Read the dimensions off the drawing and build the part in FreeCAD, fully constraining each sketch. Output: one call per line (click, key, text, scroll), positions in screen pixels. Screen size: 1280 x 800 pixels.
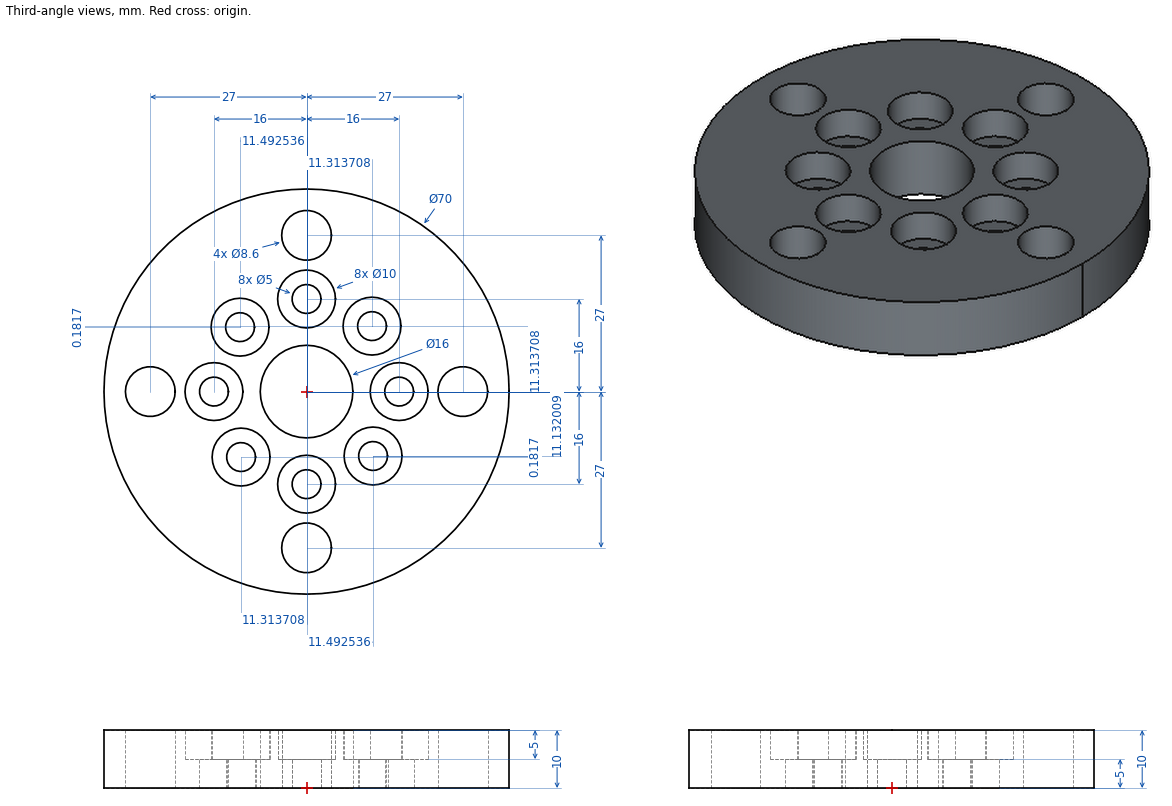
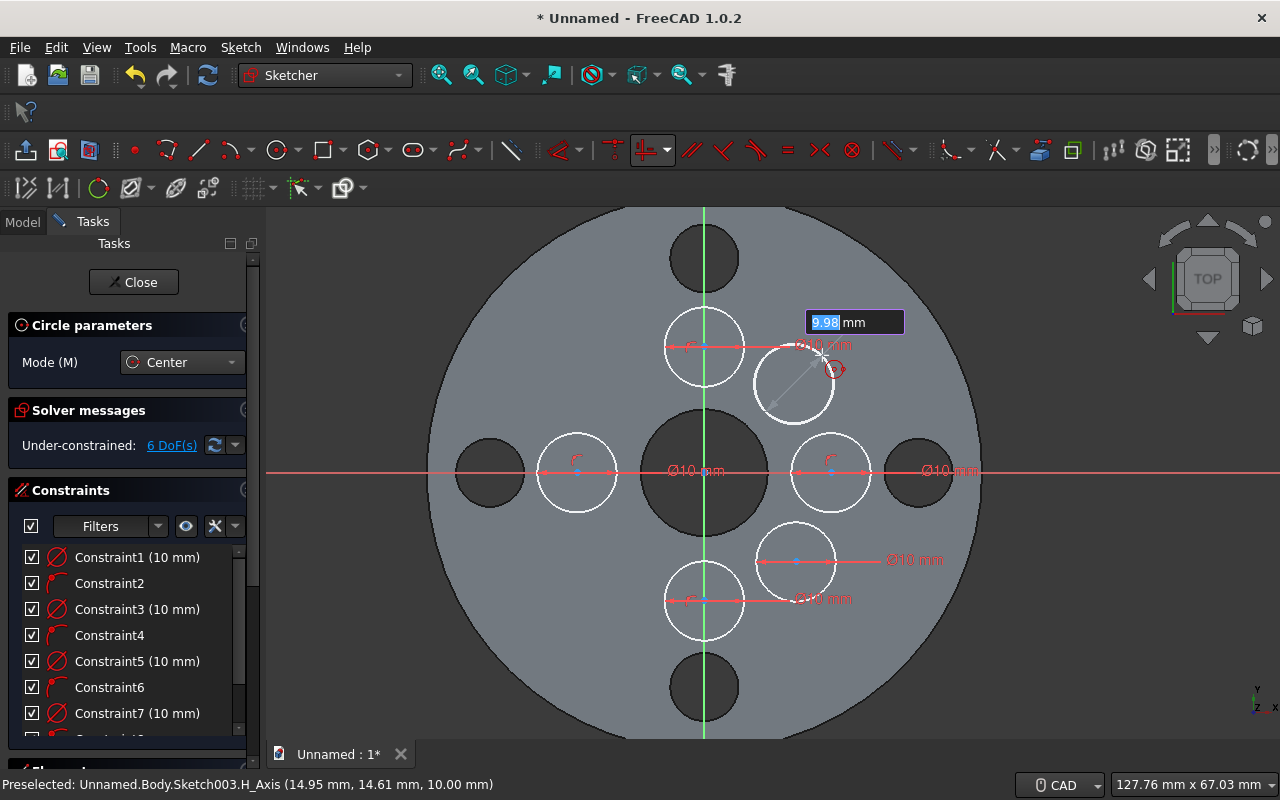
text(10)
key(Return)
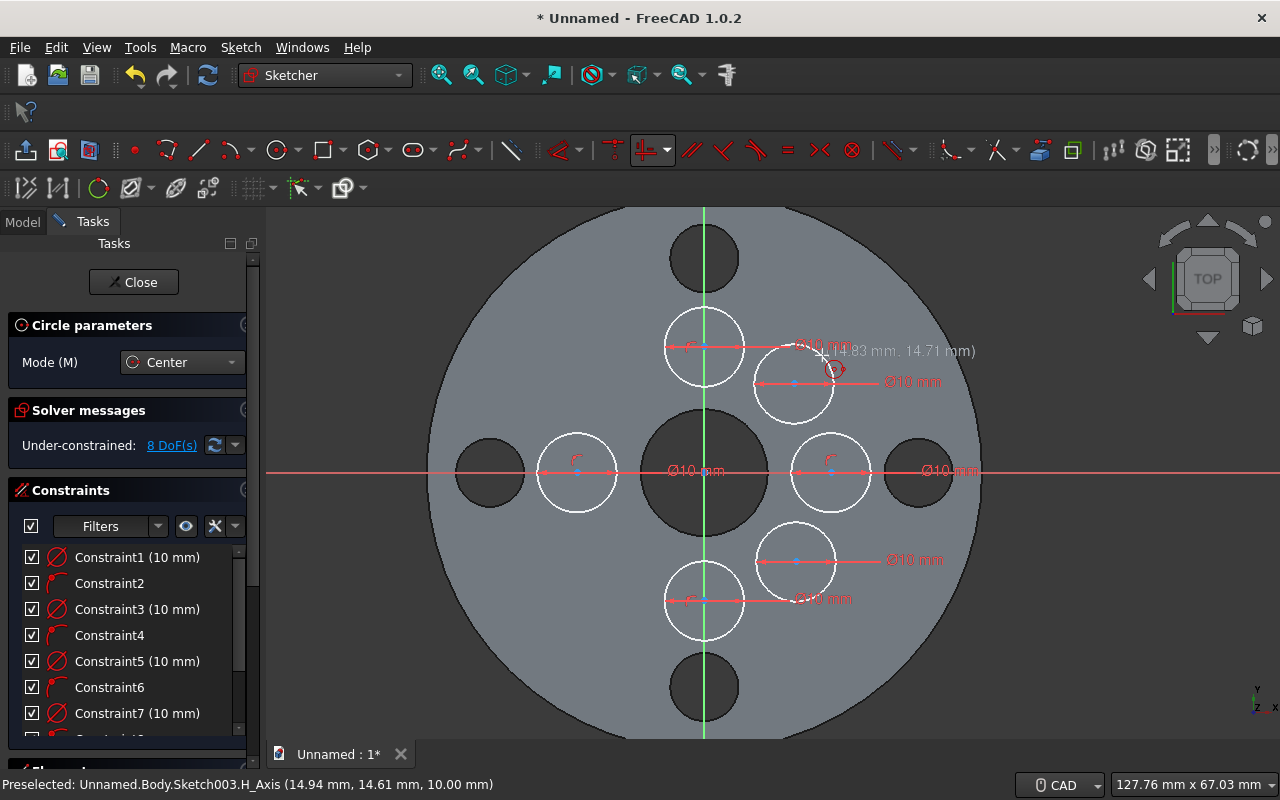
click(613, 384)
move(641, 356)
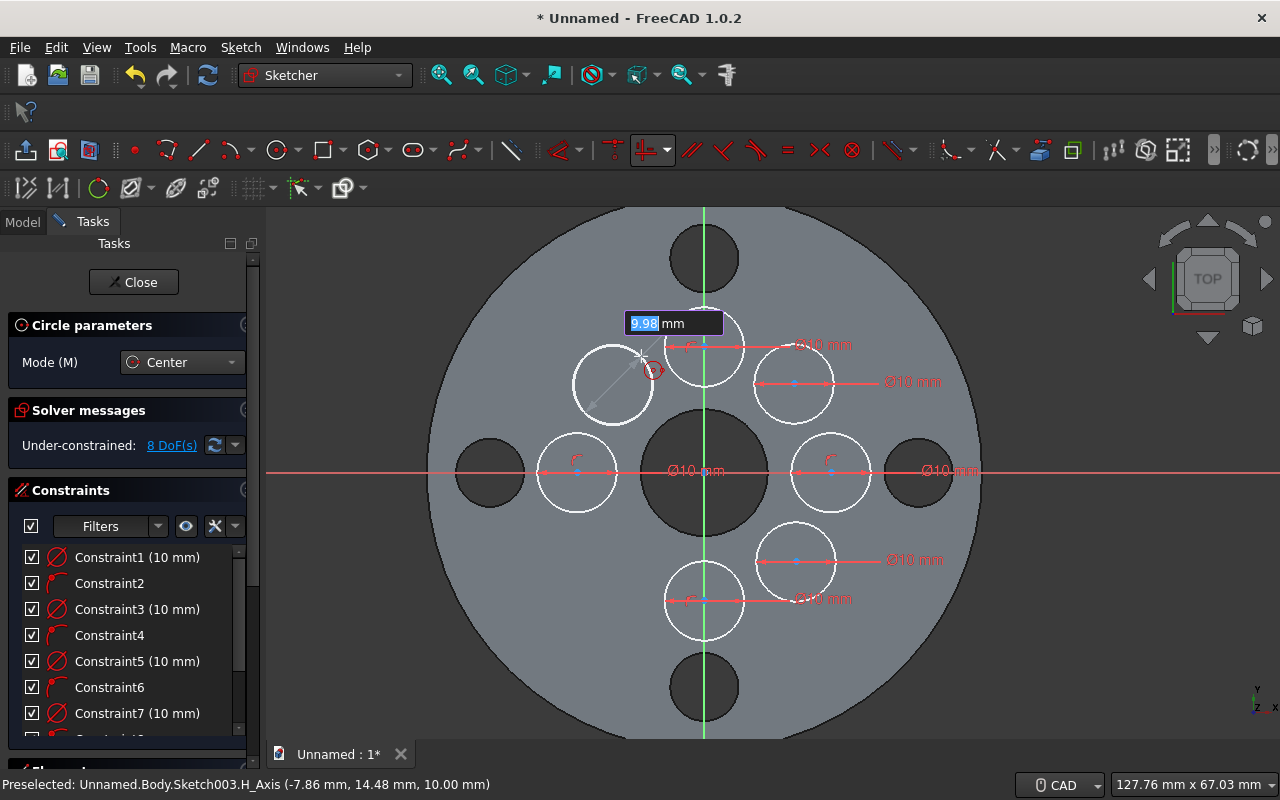
text(10)
key(Return)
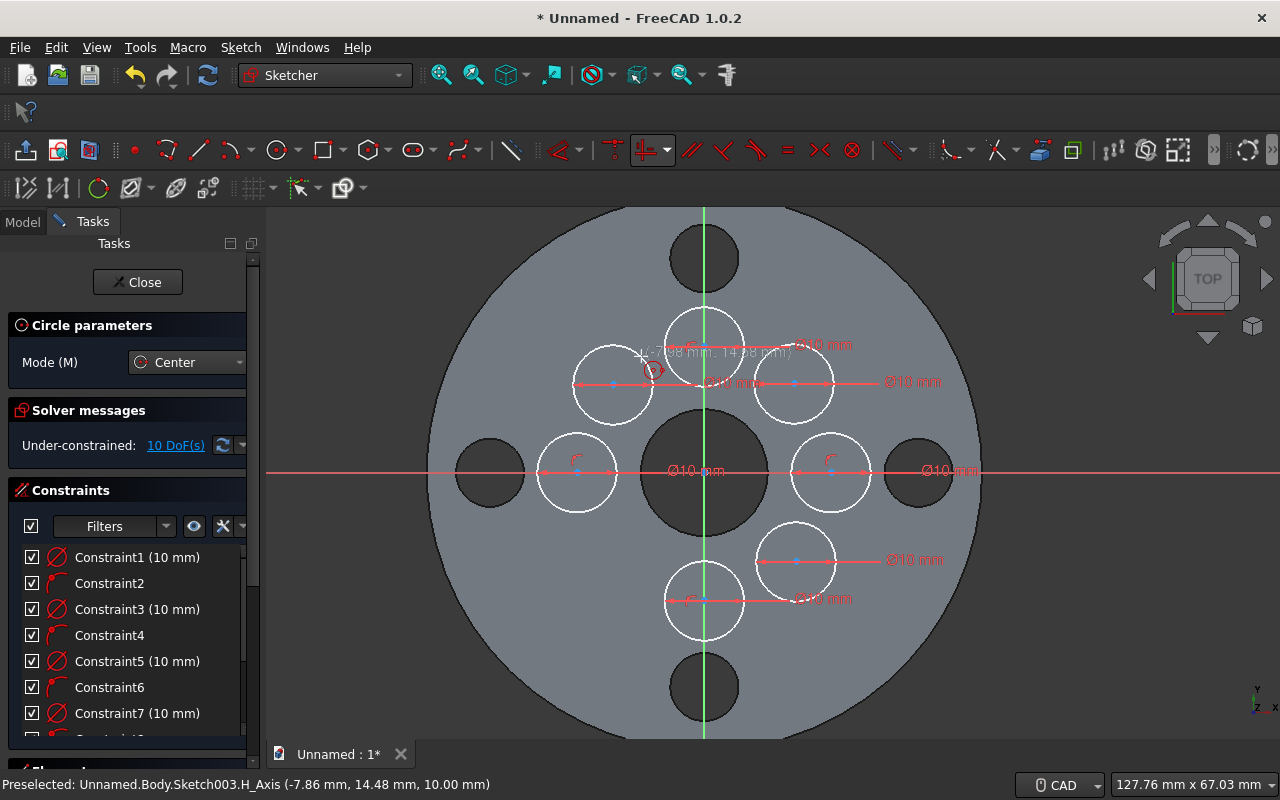
click(615, 563)
move(643, 534)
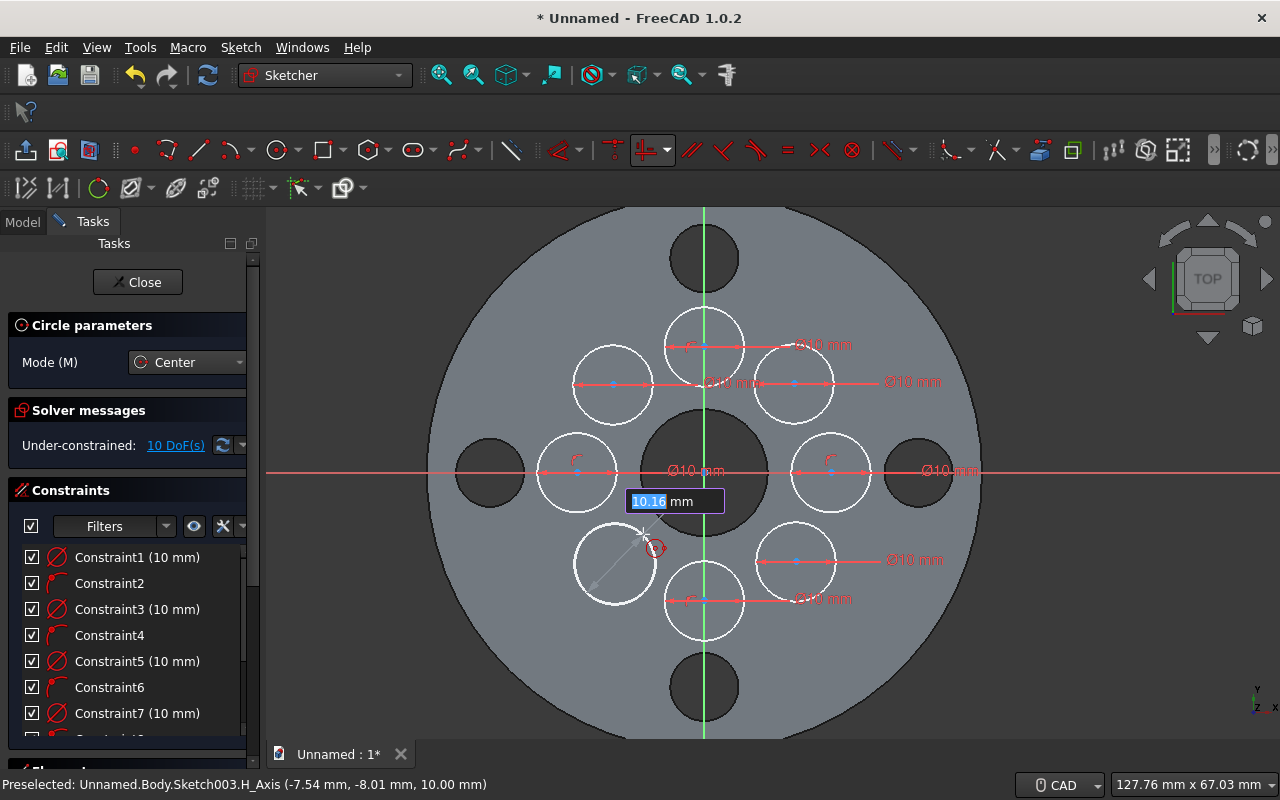
text(10)
key(Return)
key(Escape)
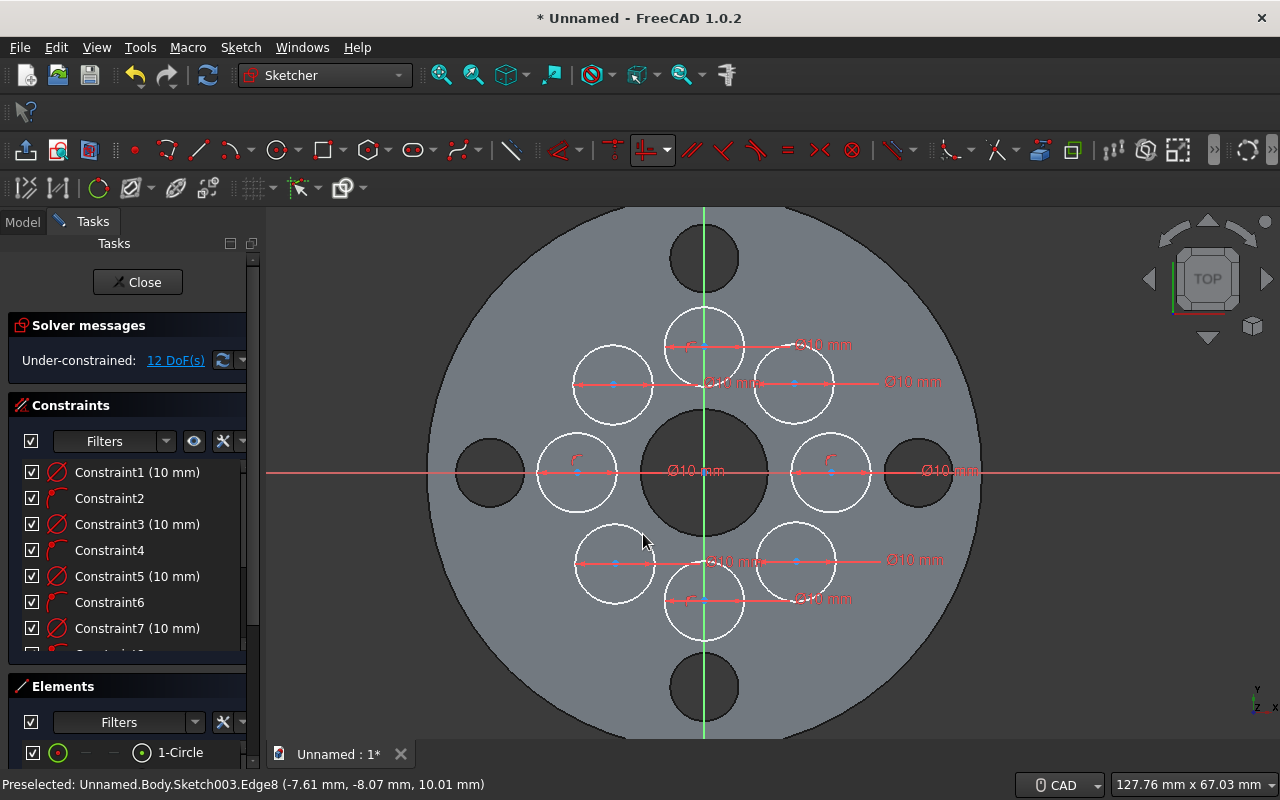
click(558, 150)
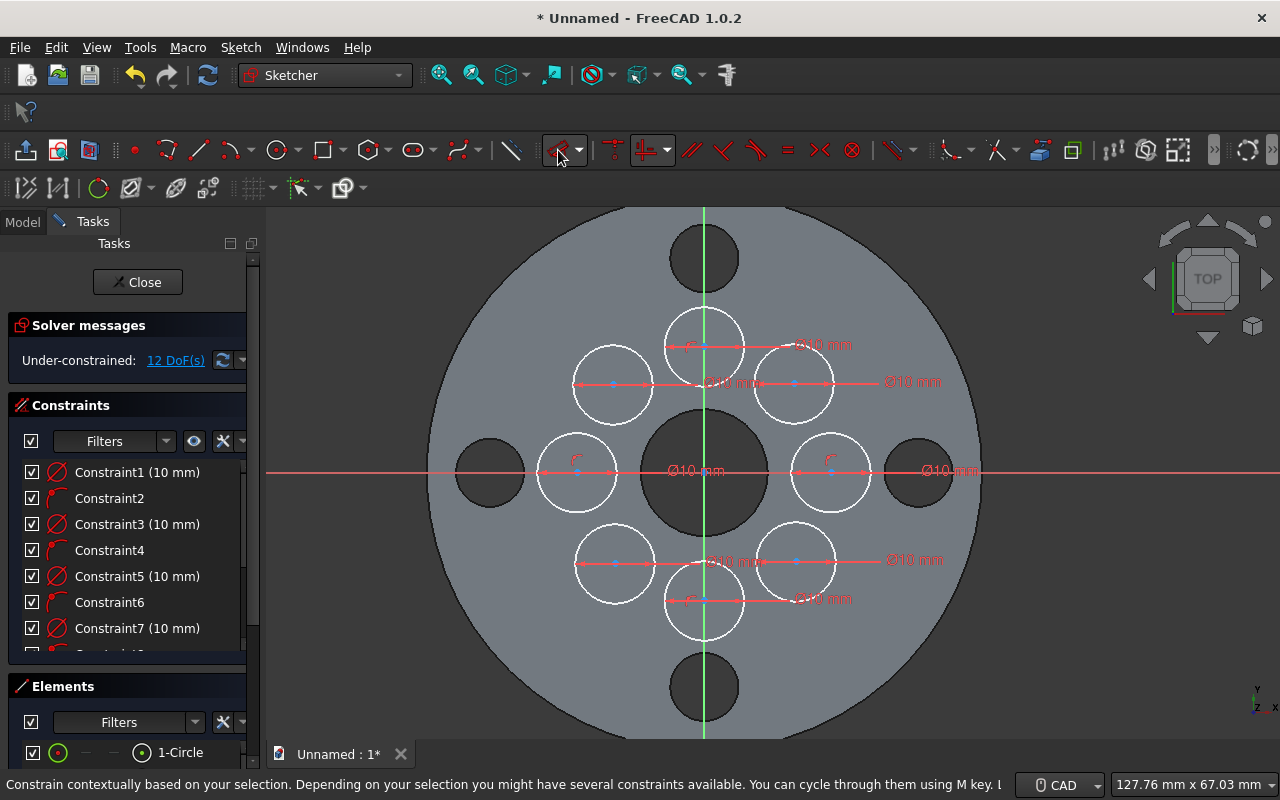
click(704, 347)
click(738, 410)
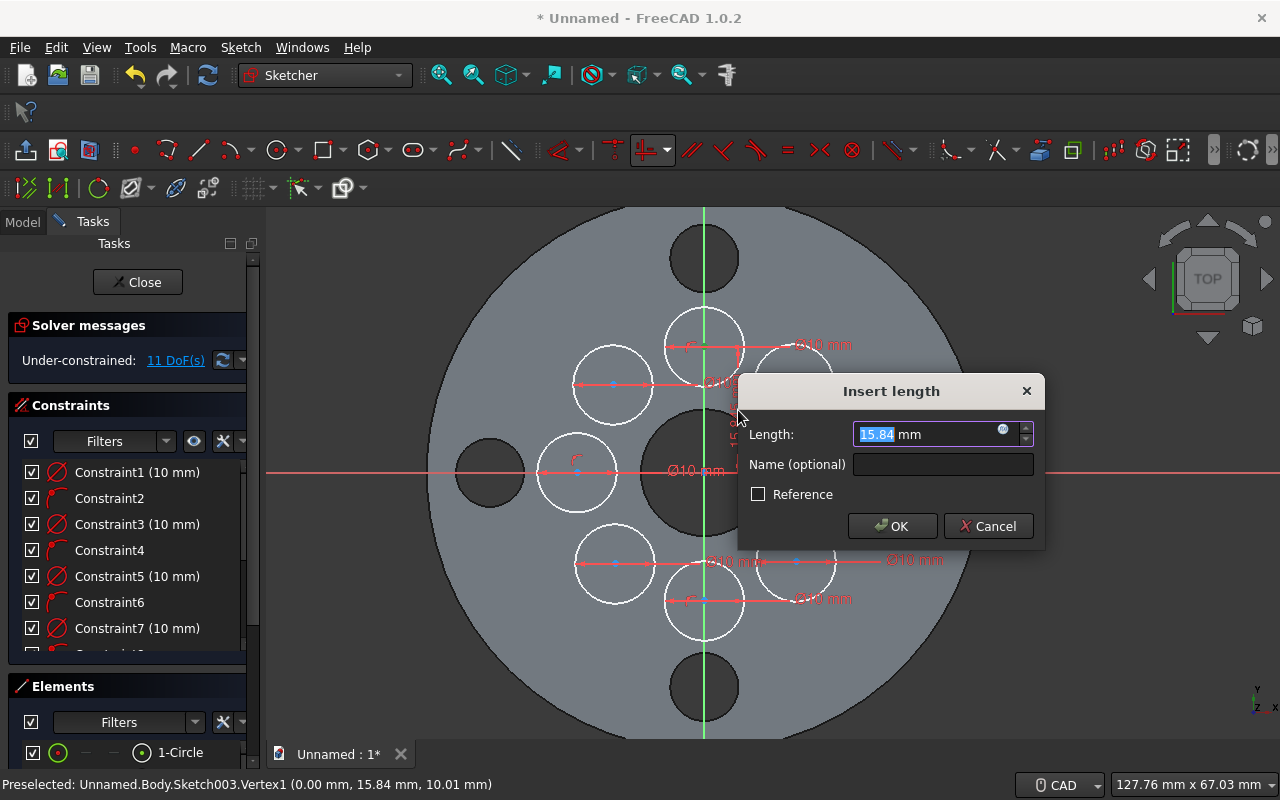
text(16)
key(Return)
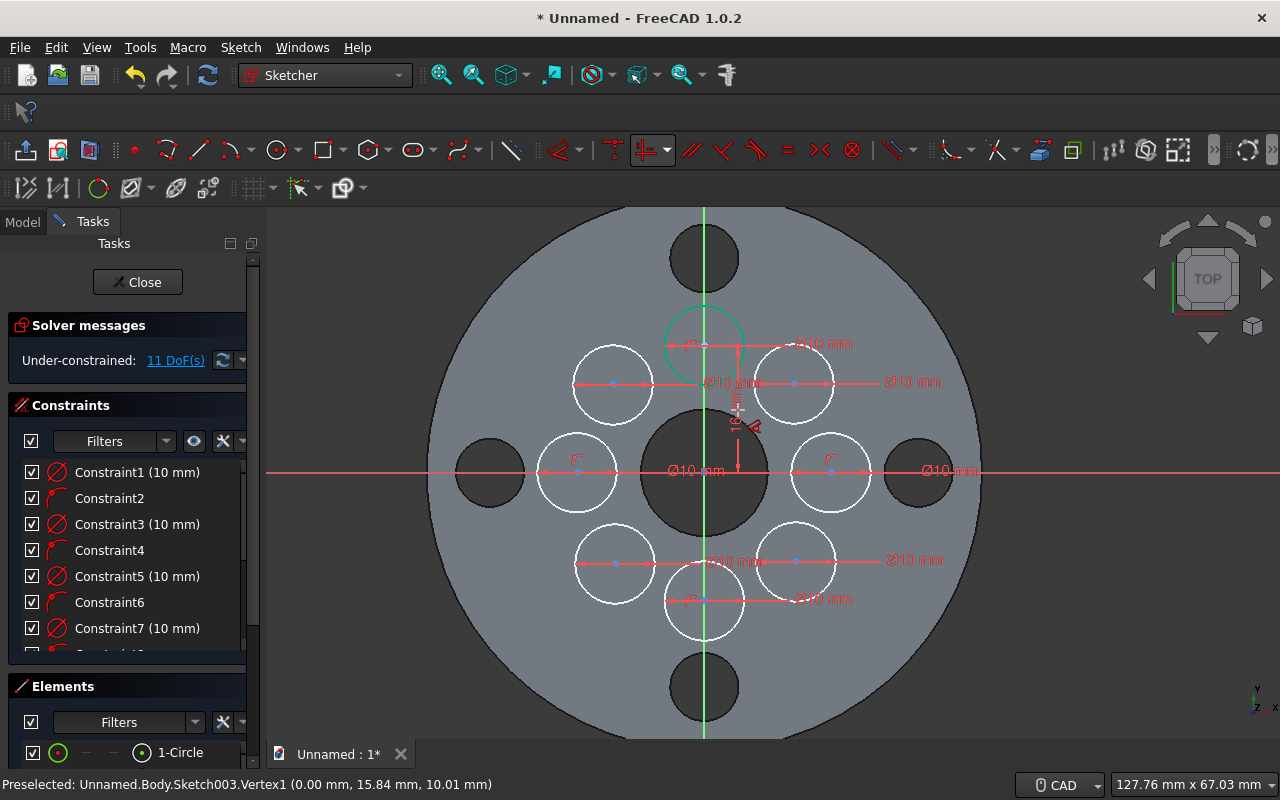
click(831, 473)
click(768, 507)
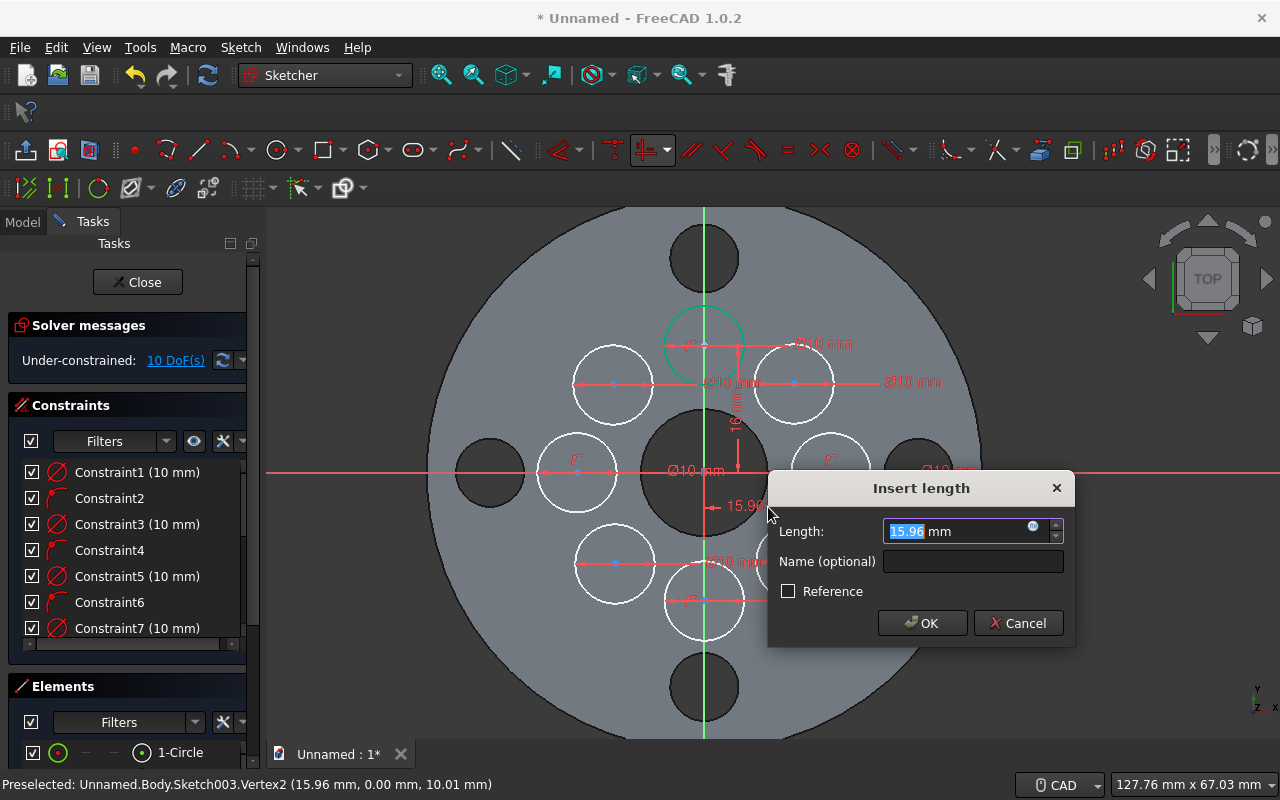
text(16)
key(Return)